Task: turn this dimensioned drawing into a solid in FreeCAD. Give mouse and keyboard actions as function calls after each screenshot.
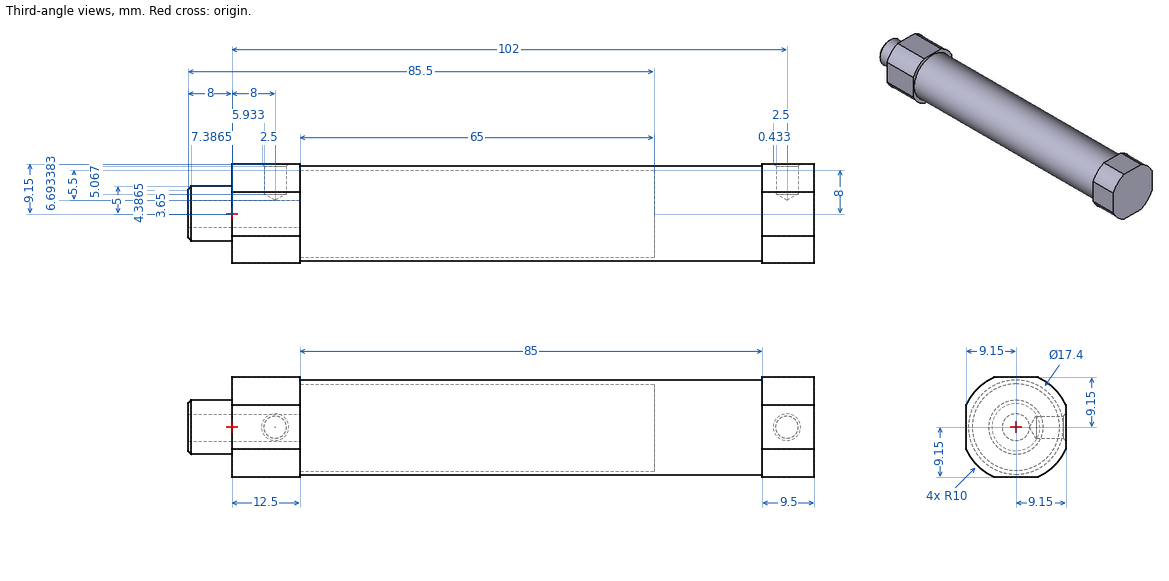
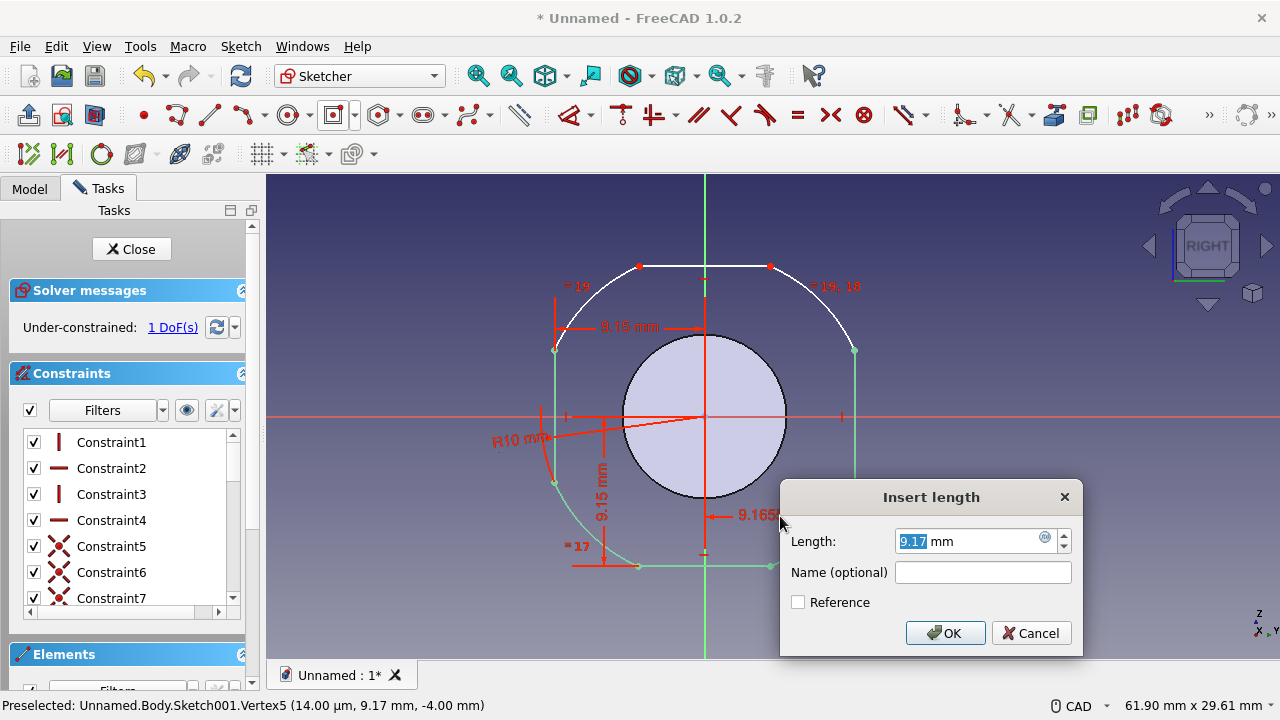
text(9.15)
key(Return)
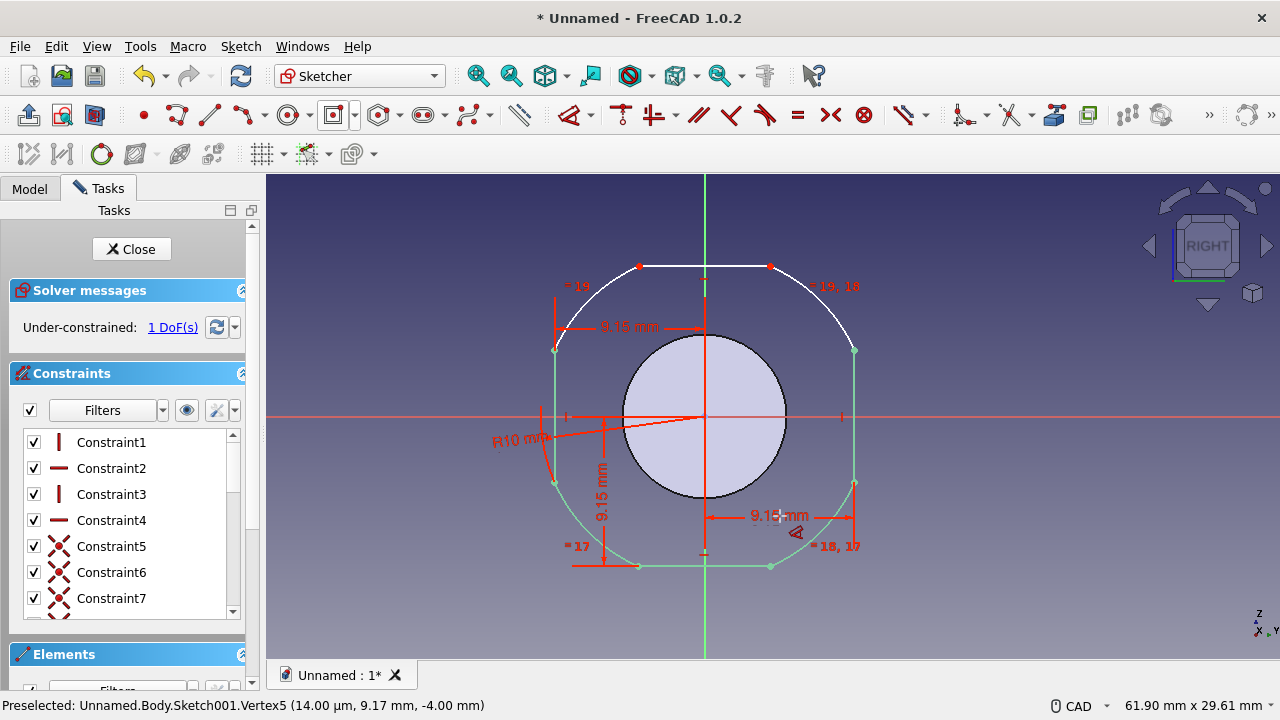
click(770, 266)
click(804, 341)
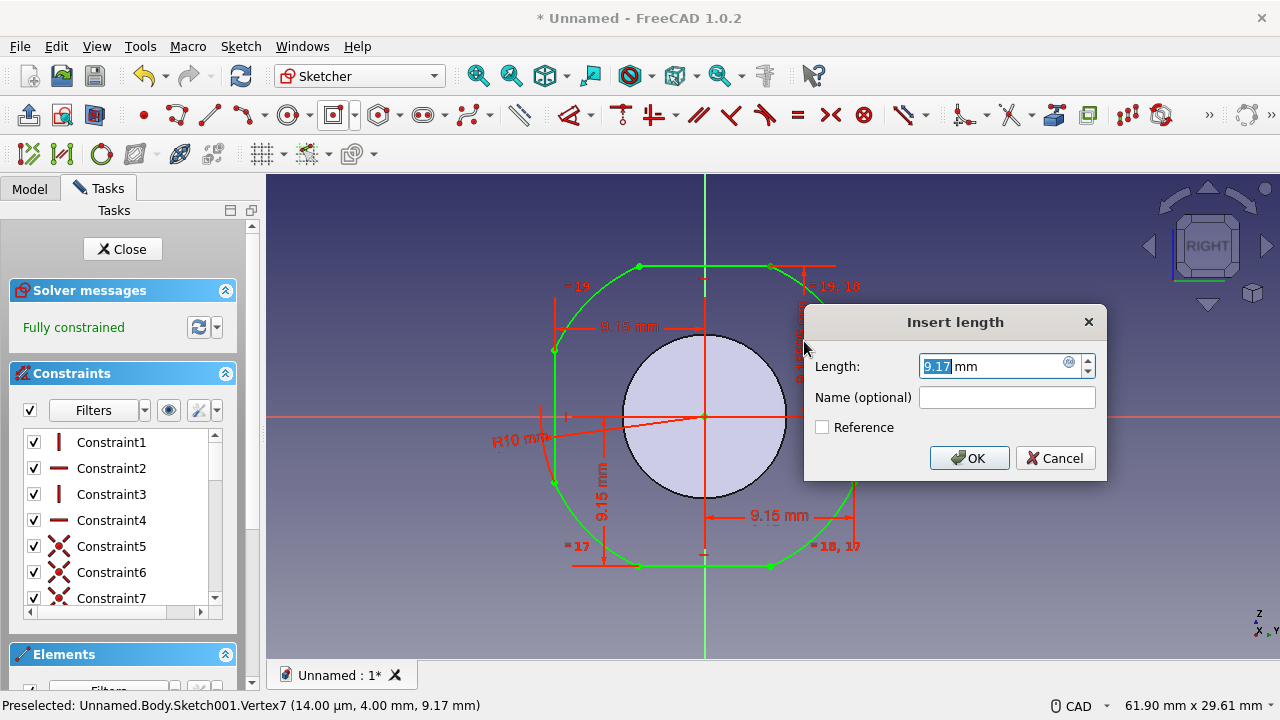
text(9.15)
key(Return)
key(Escape)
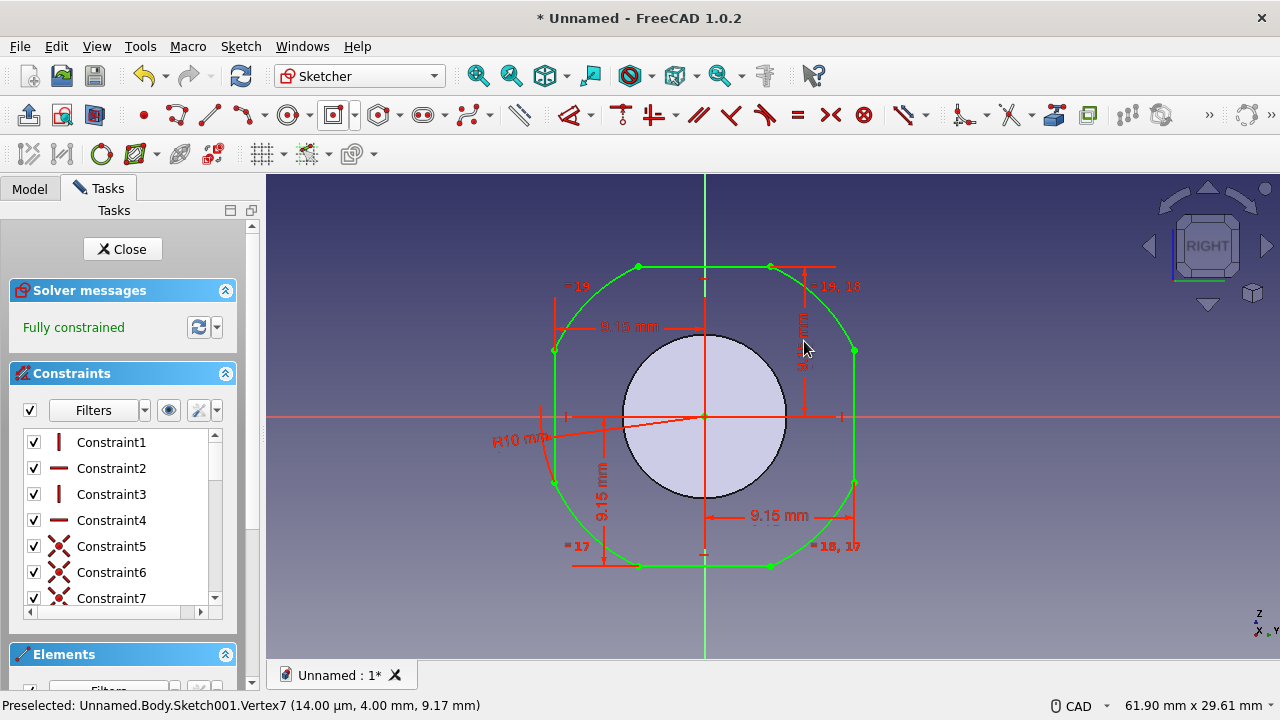
click(123, 249)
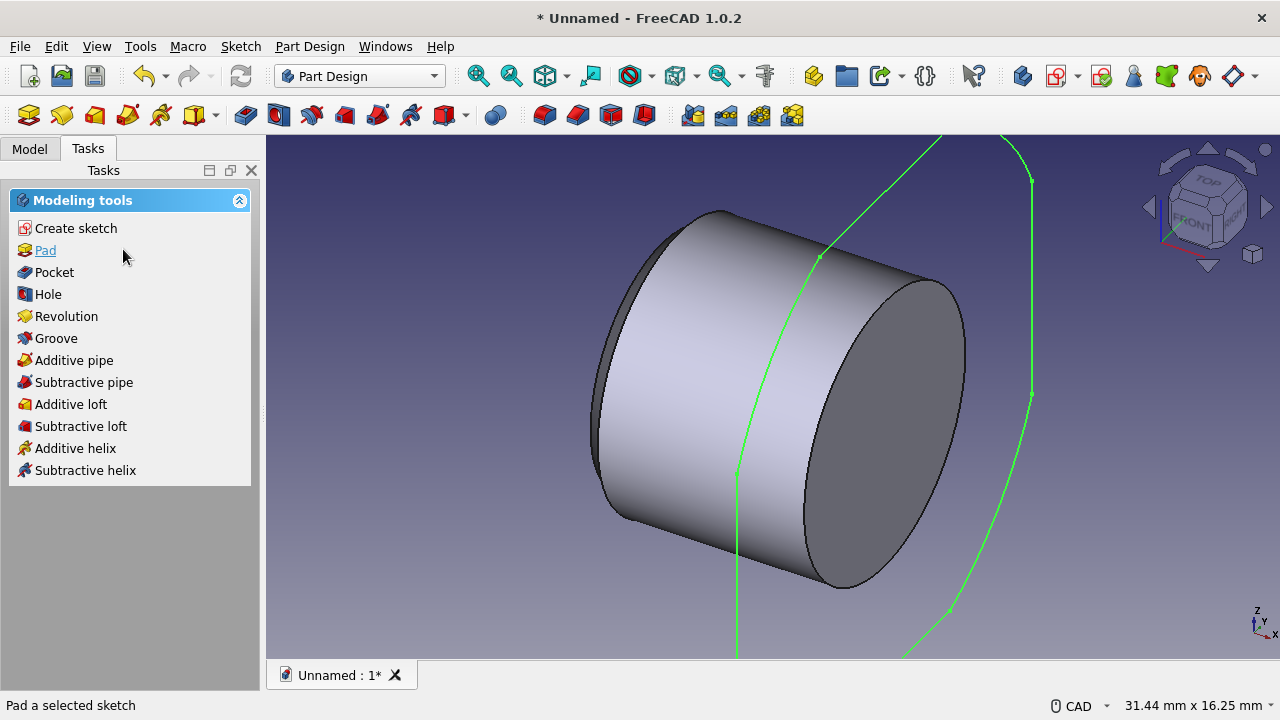
click(29, 116)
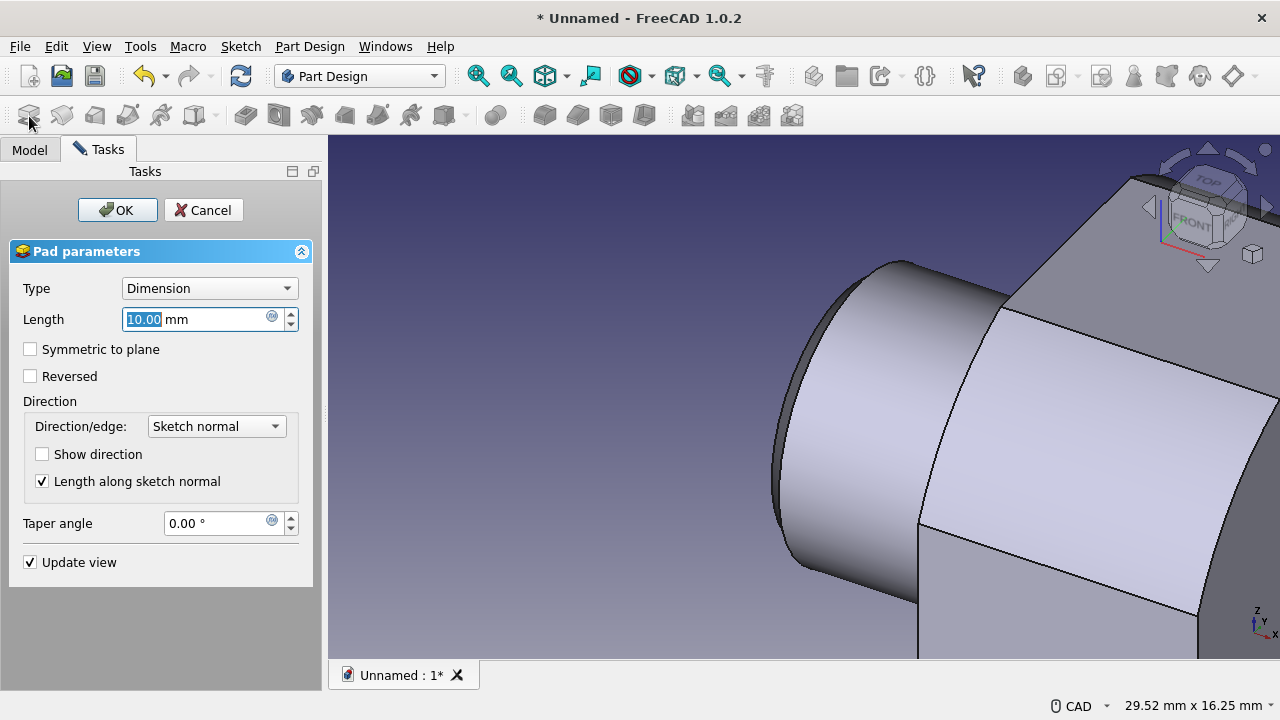
text(12.5)
key(Tab)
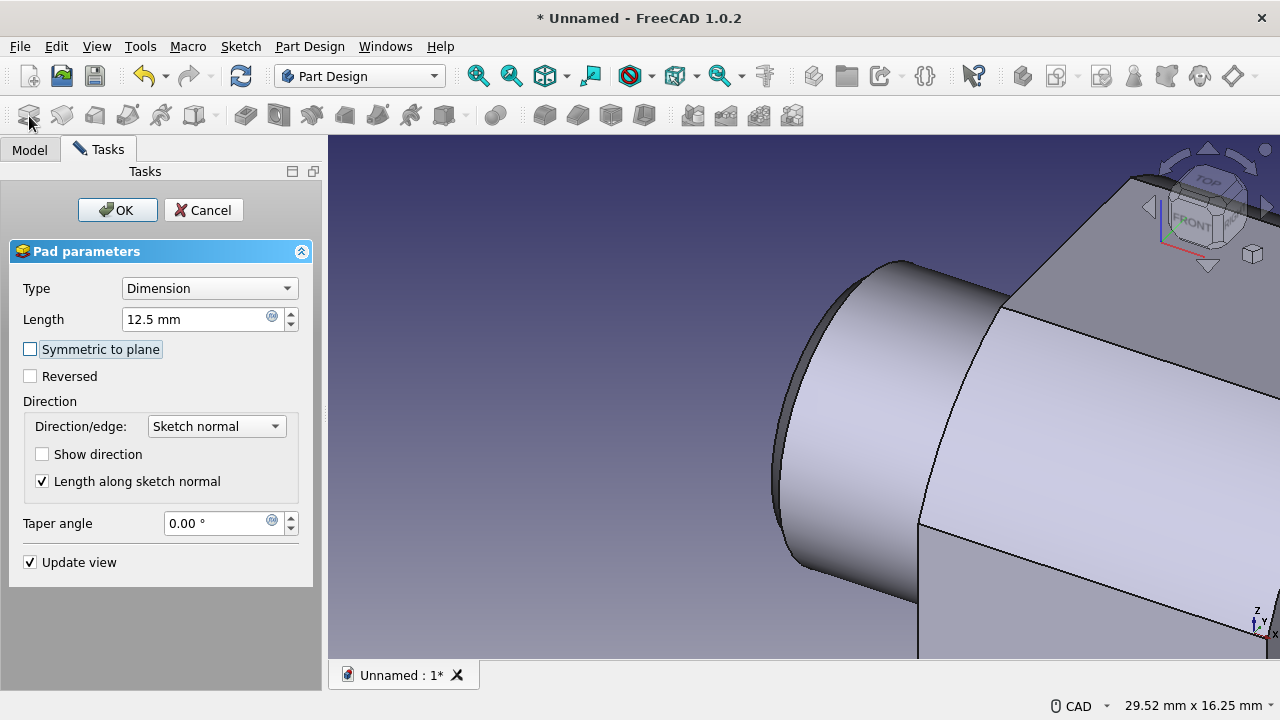
click(118, 210)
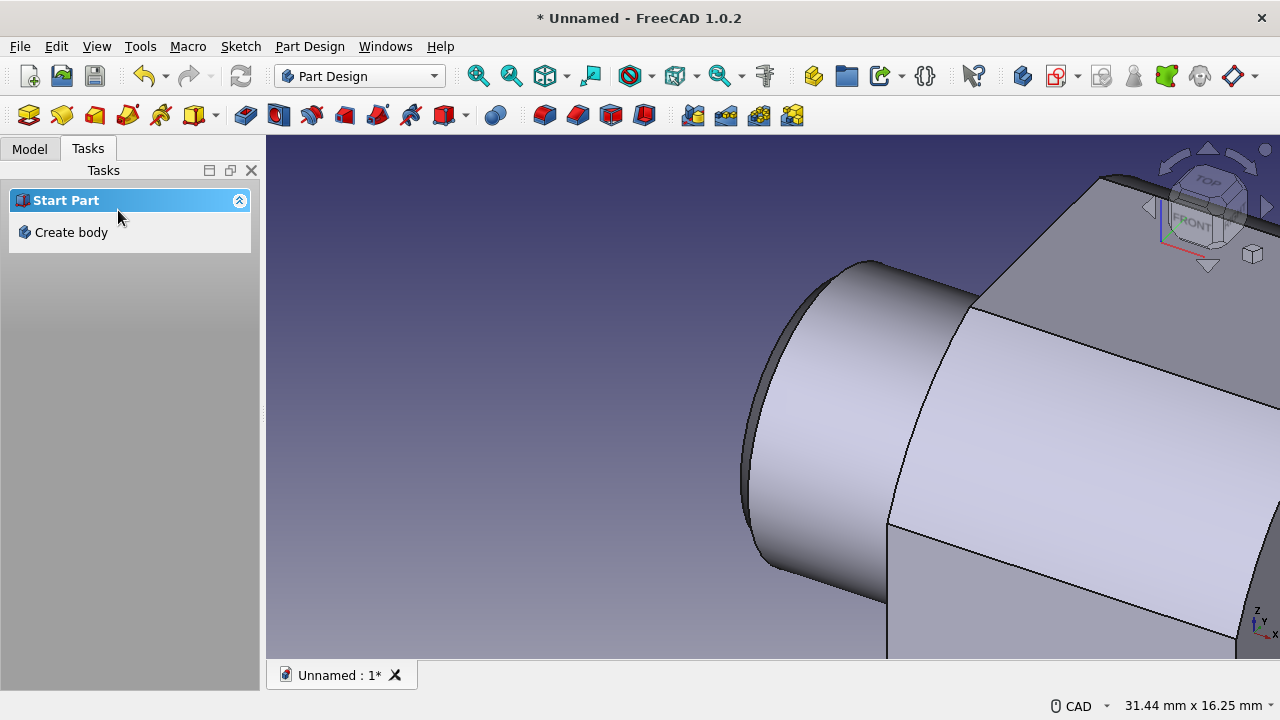
click(479, 76)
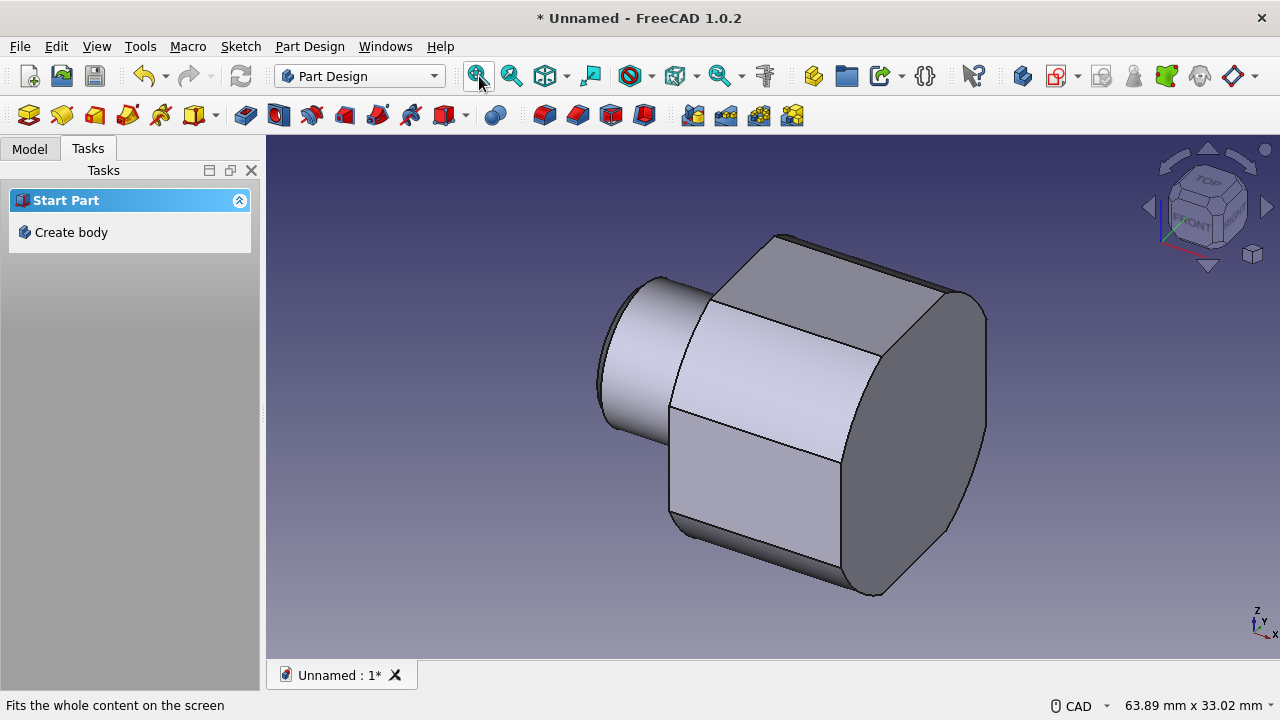
click(914, 443)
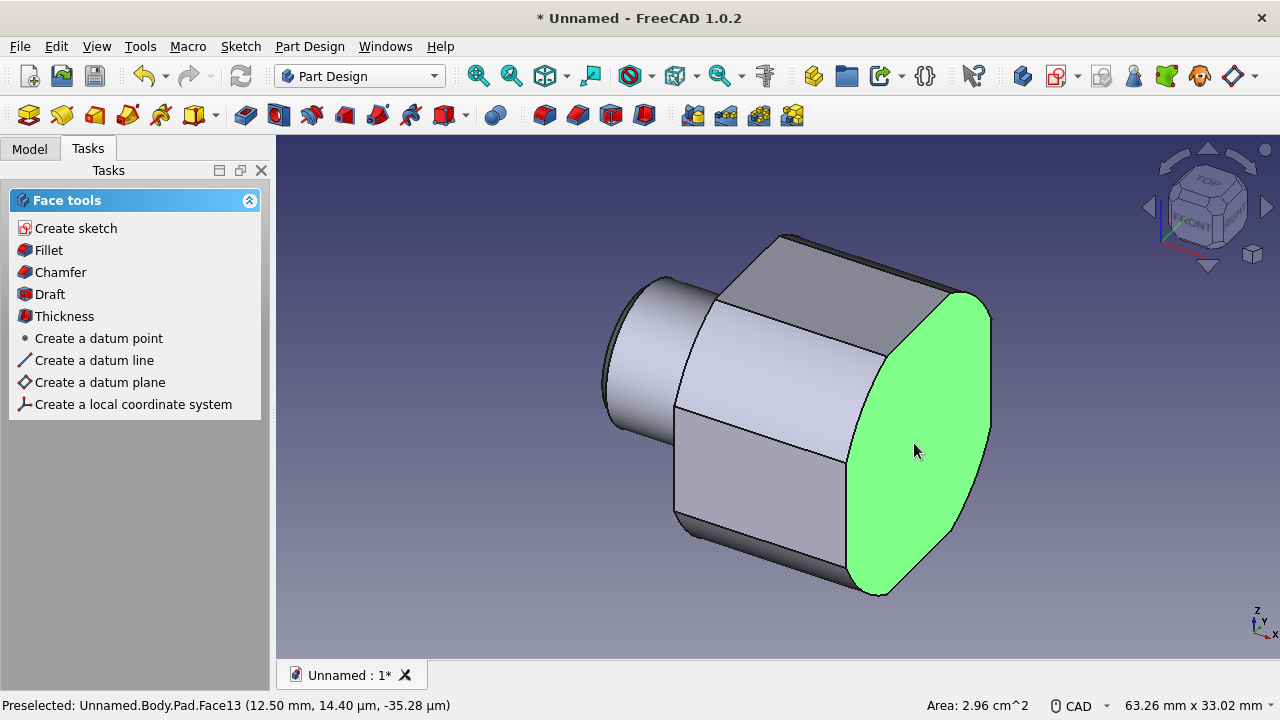
click(1056, 76)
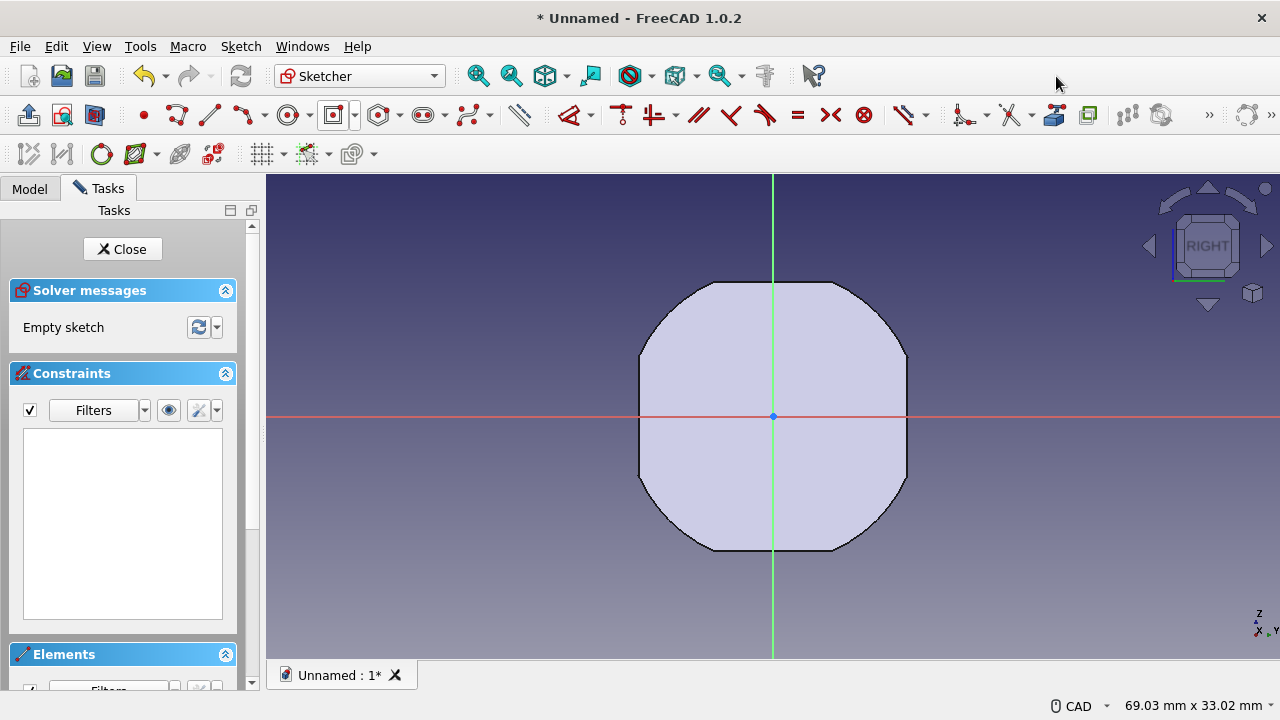
click(288, 116)